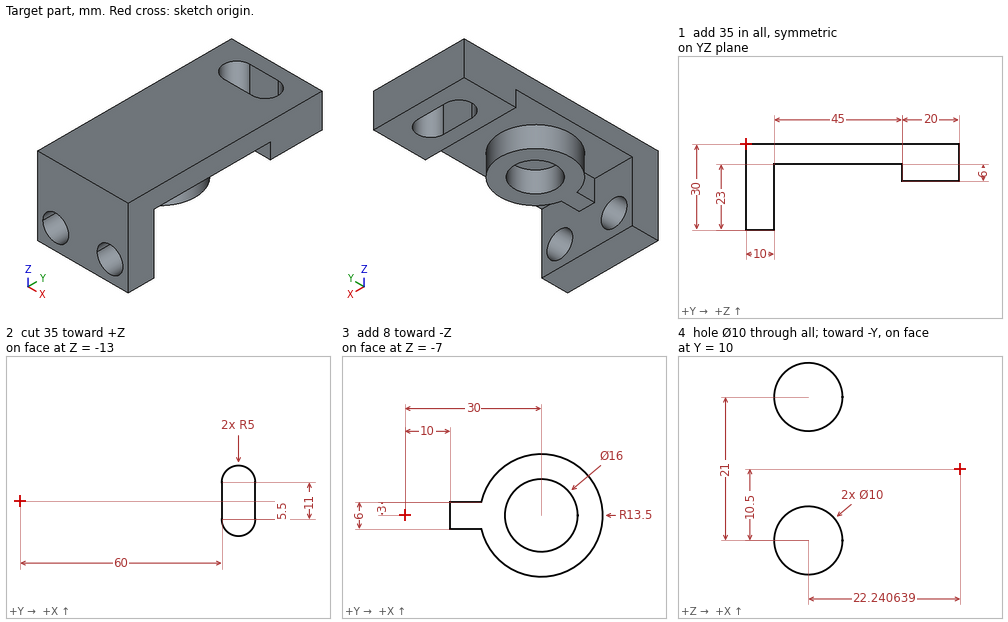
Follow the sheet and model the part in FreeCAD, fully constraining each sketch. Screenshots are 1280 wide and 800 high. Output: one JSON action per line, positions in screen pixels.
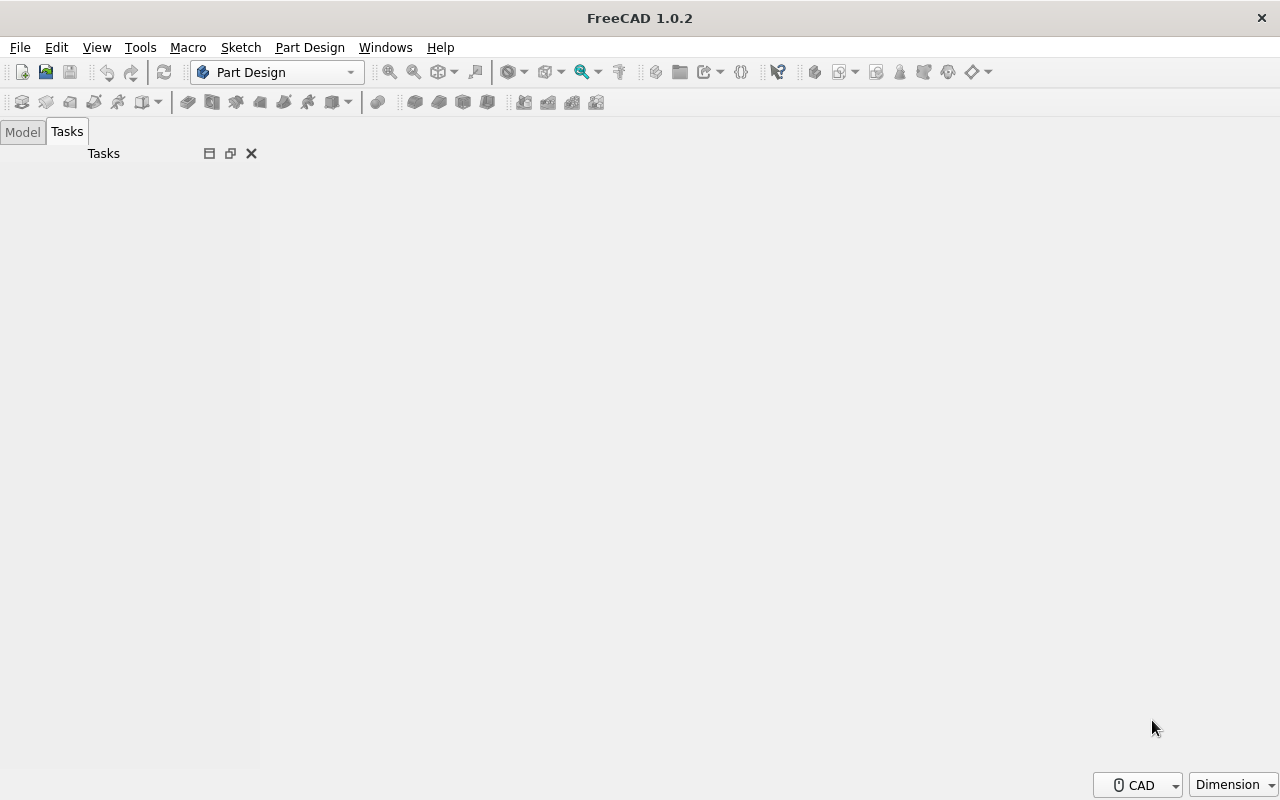
{"action": "left_click", "coordinate": [22, 72]}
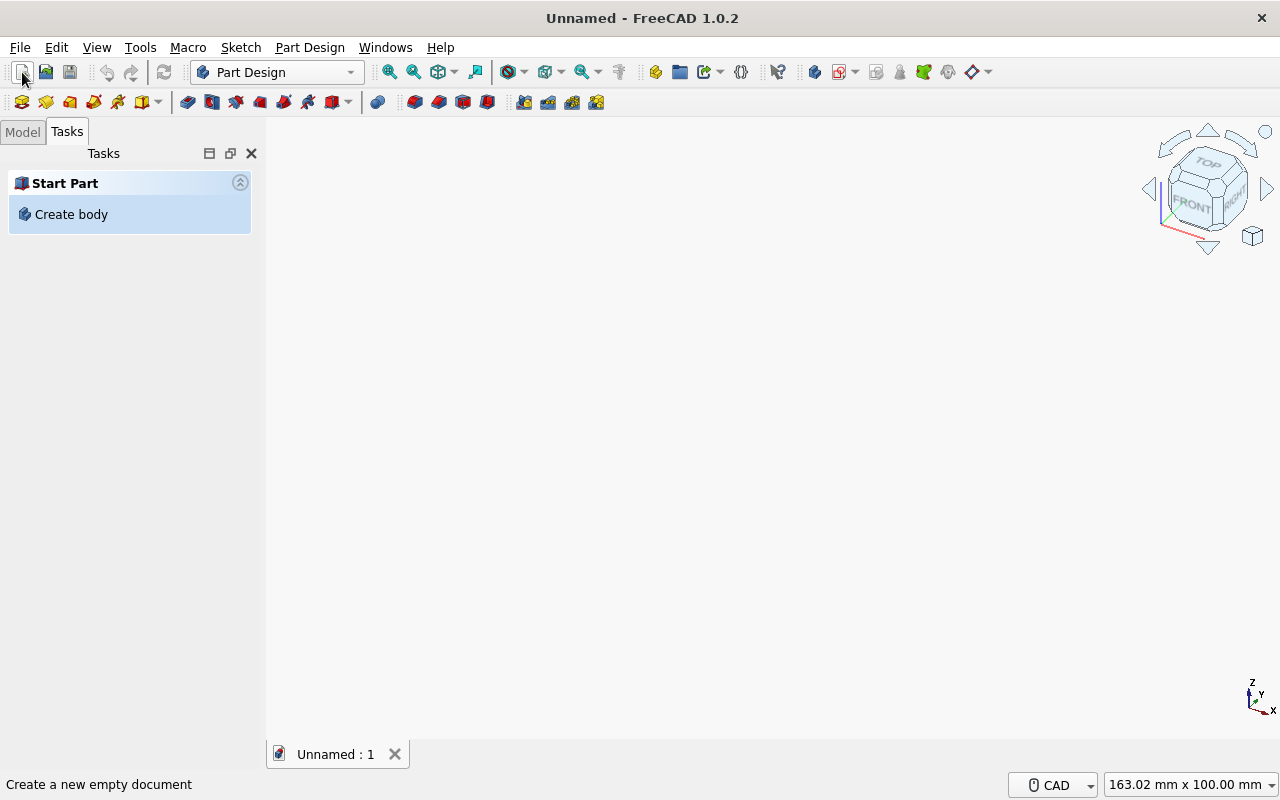
{"action": "left_click", "coordinate": [840, 72]}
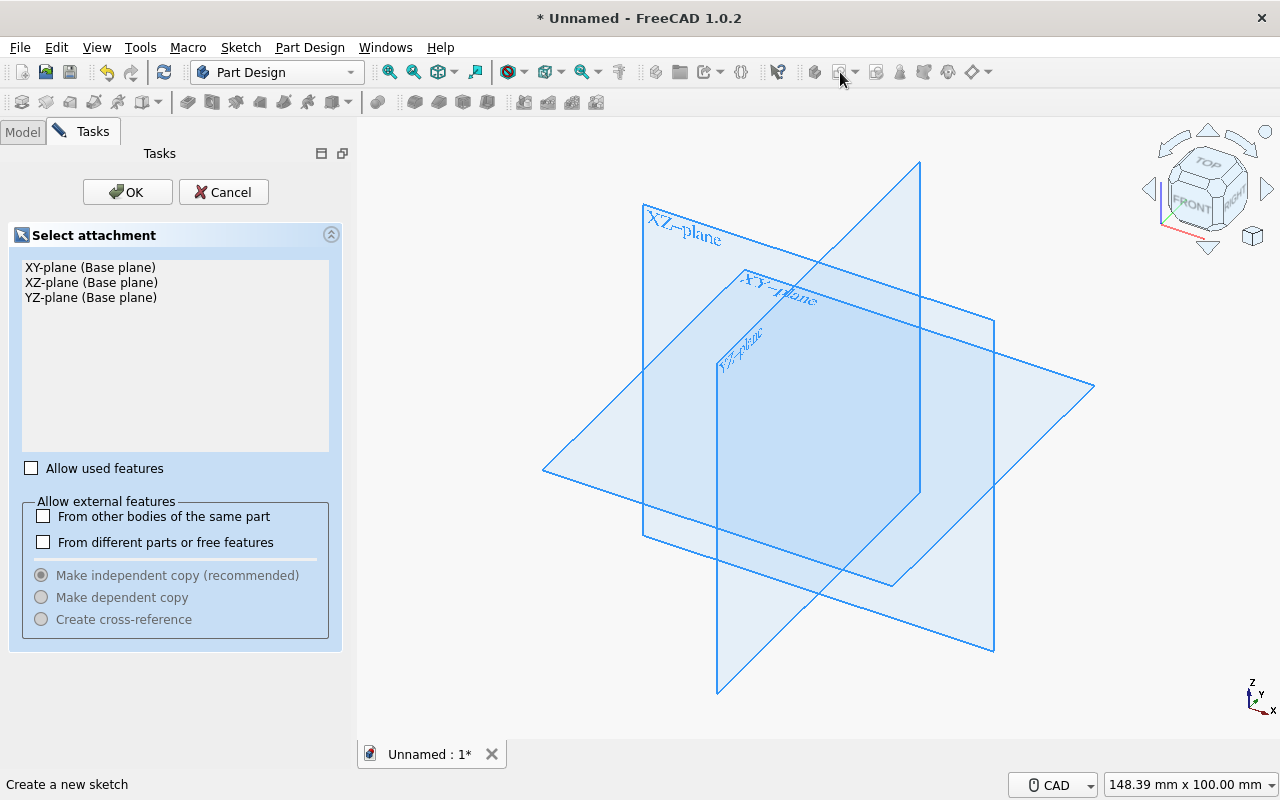
{"action": "left_click", "coordinate": [82, 298]}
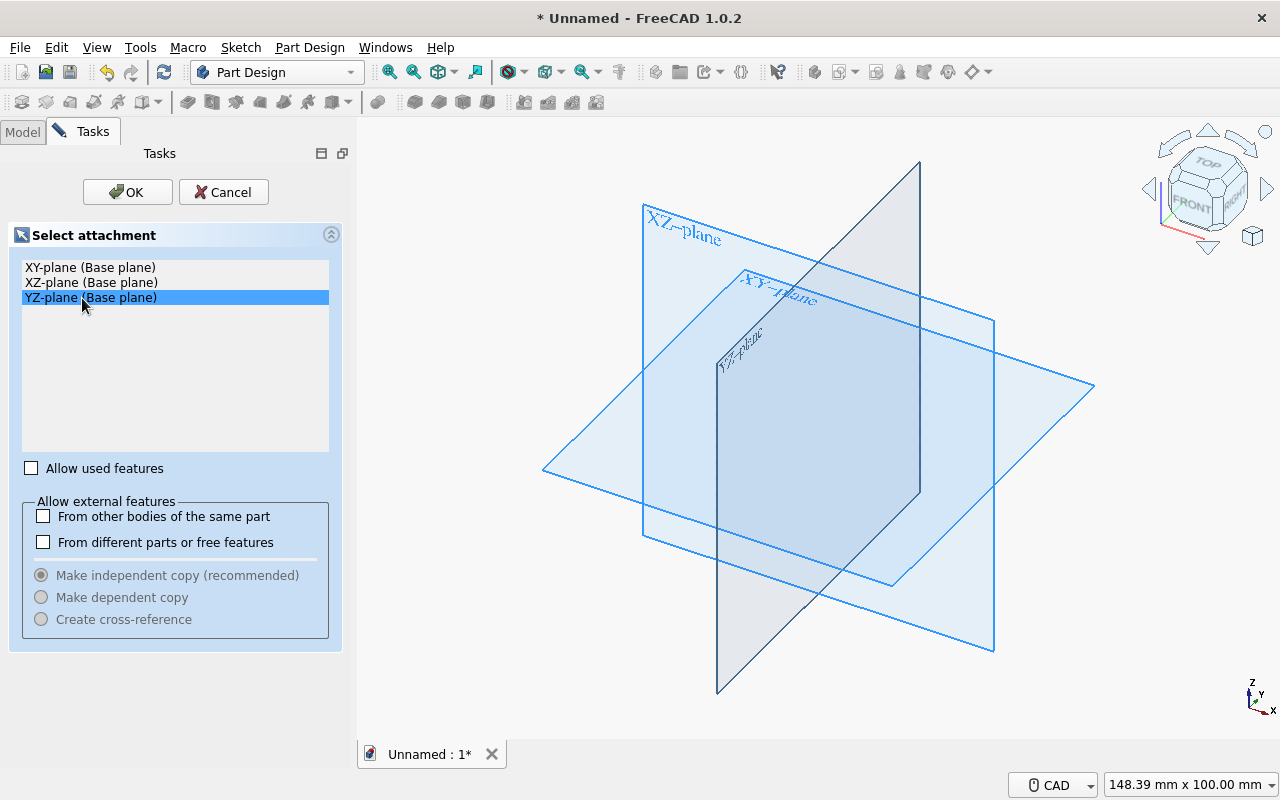
{"action": "left_click", "coordinate": [128, 192]}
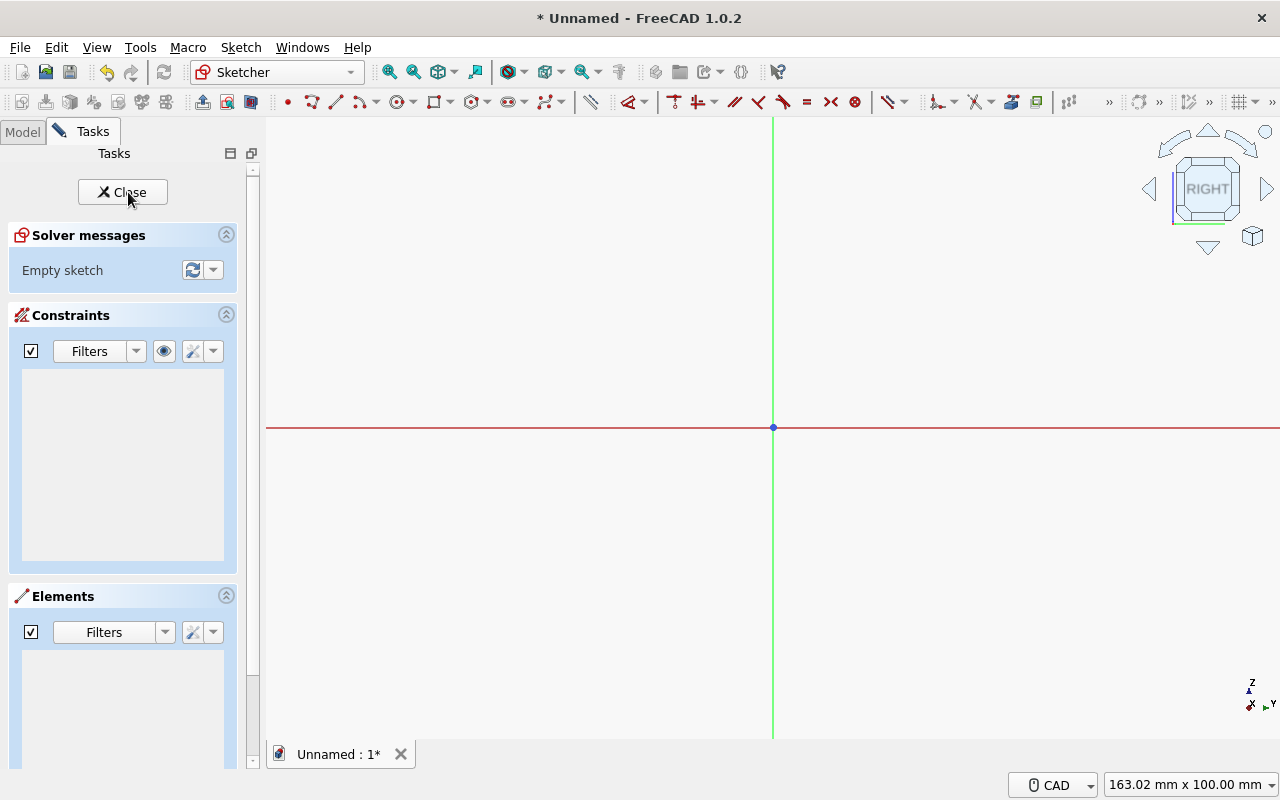
{"action": "scroll", "coordinate": [294, 145], "scroll_direction": "down", "scroll_amount": 1}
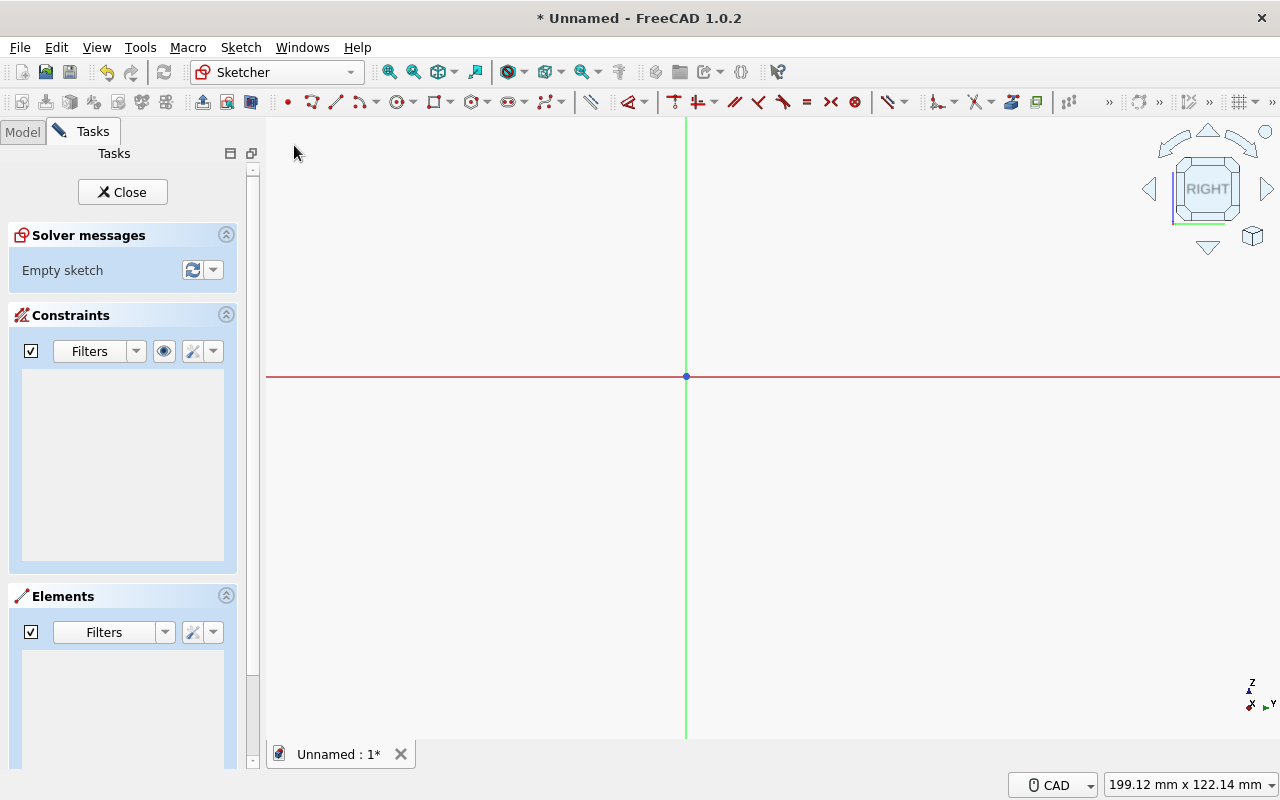
{"action": "scroll", "coordinate": [1115, 504], "scroll_direction": "up", "scroll_amount": 2}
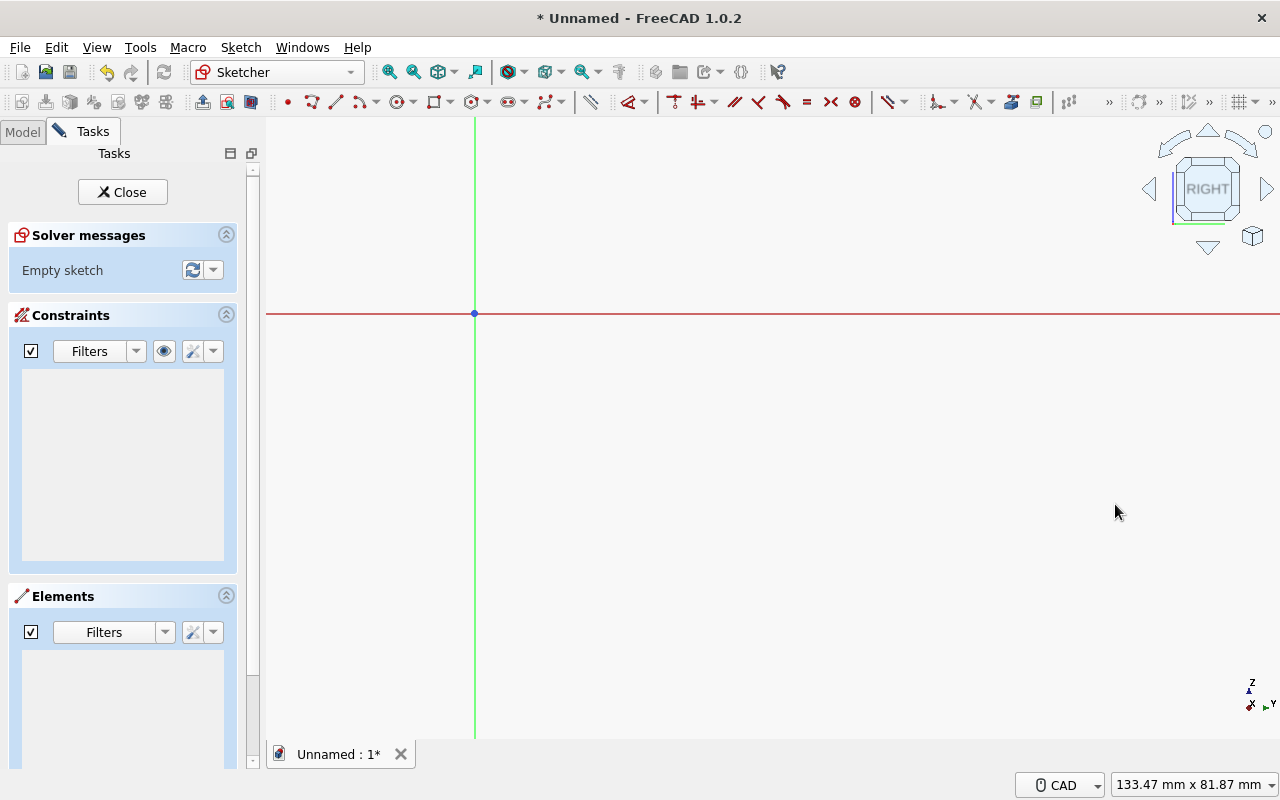
{"action": "left_click", "coordinate": [312, 102]}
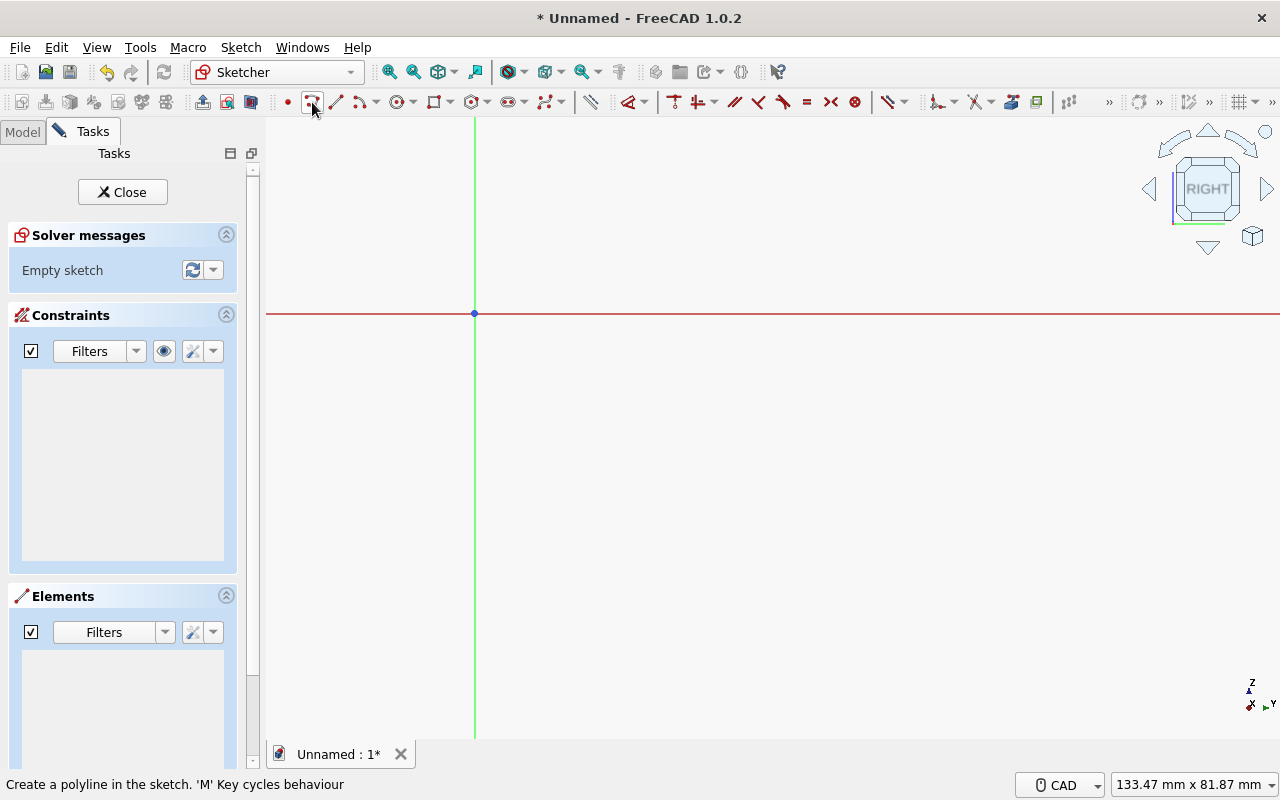
{"action": "left_click", "coordinate": [475, 314]}
{"action": "left_click", "coordinate": [484, 542]}
{"action": "left_click", "coordinate": [551, 542]}
{"action": "left_click", "coordinate": [551, 367]}
{"action": "left_click", "coordinate": [893, 367]}
{"action": "left_click", "coordinate": [893, 413]}
{"action": "left_click", "coordinate": [1045, 413]}
{"action": "left_click", "coordinate": [1045, 323]}
{"action": "left_click", "coordinate": [475, 314]}
{"action": "key", "text": "Escape"}
{"action": "key", "text": "Escape"}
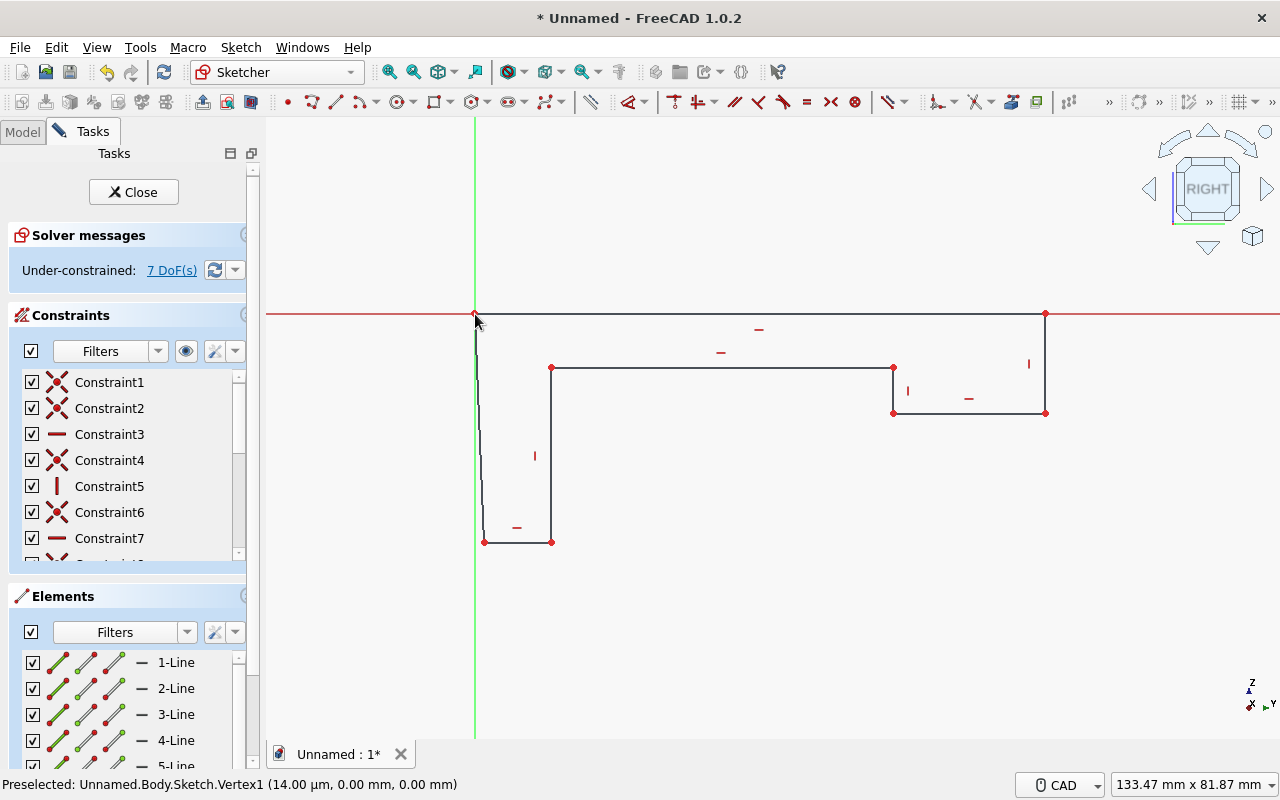
{"action": "left_click", "coordinate": [478, 383]}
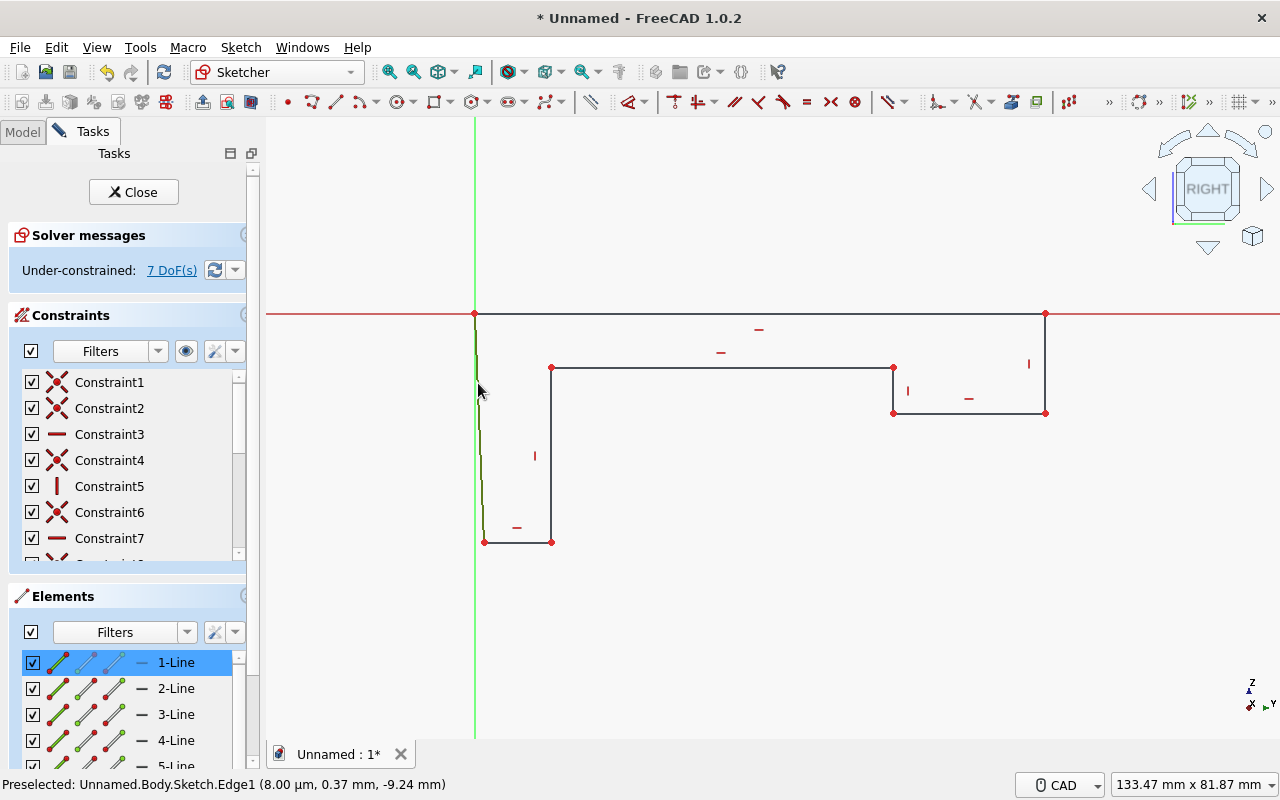
{"action": "key", "text": "v"}